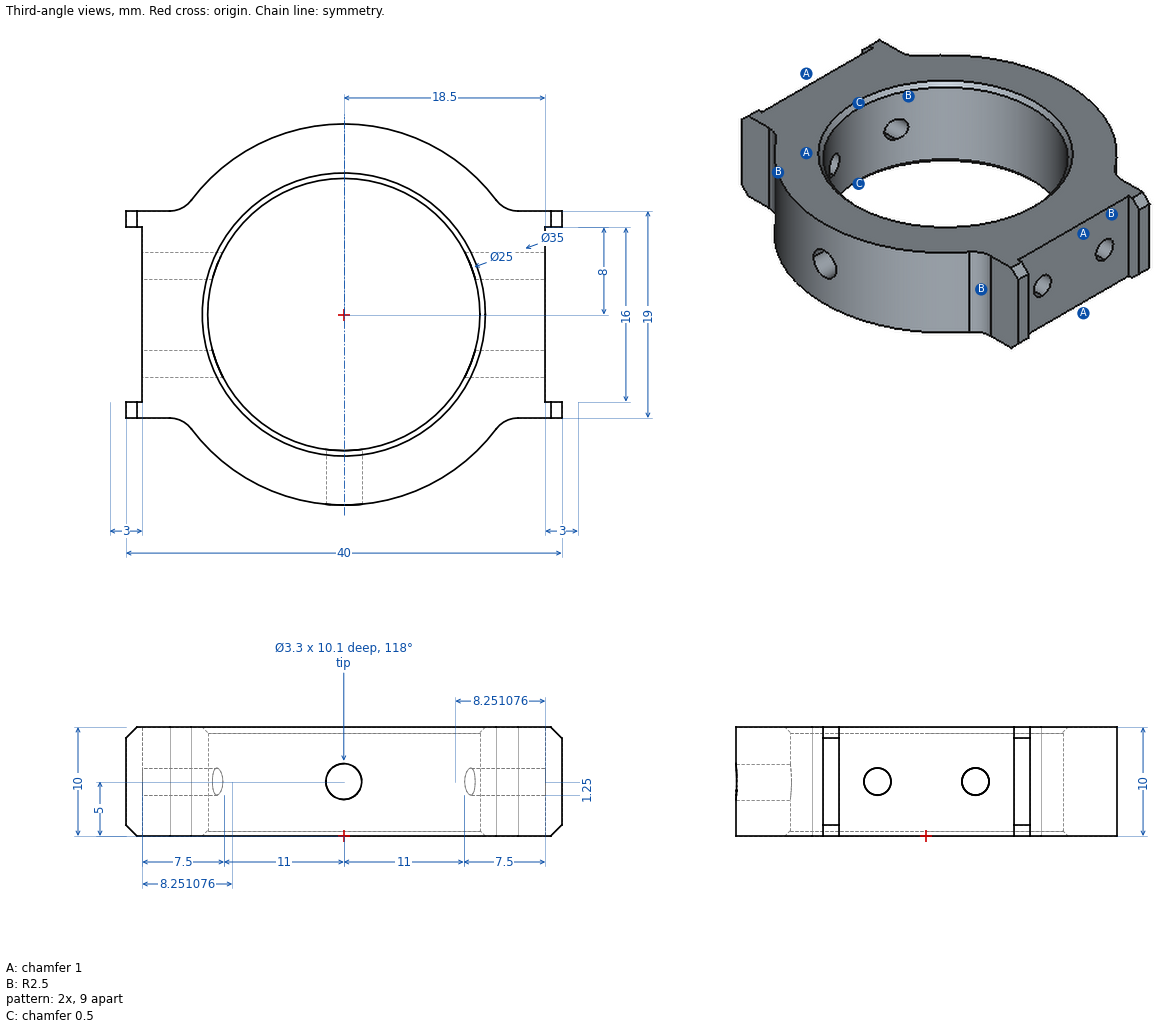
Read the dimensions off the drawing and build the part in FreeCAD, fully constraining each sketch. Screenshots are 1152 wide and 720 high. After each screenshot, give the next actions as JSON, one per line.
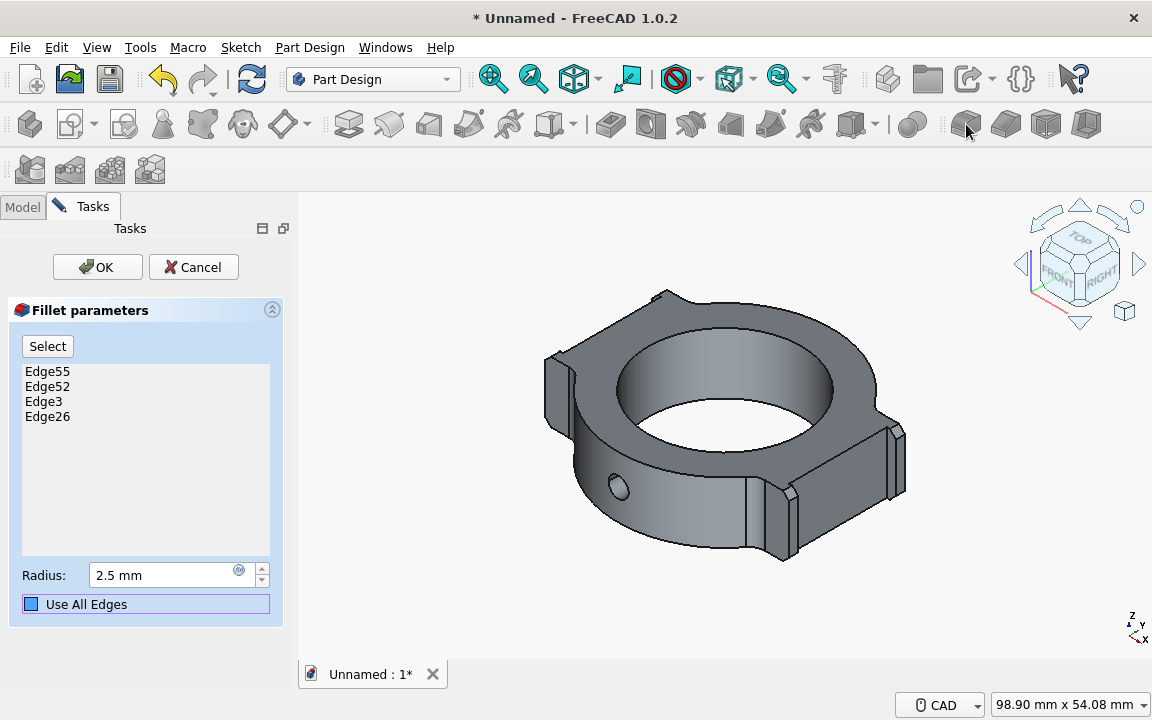
{"action": "left_click", "coordinate": [98, 267]}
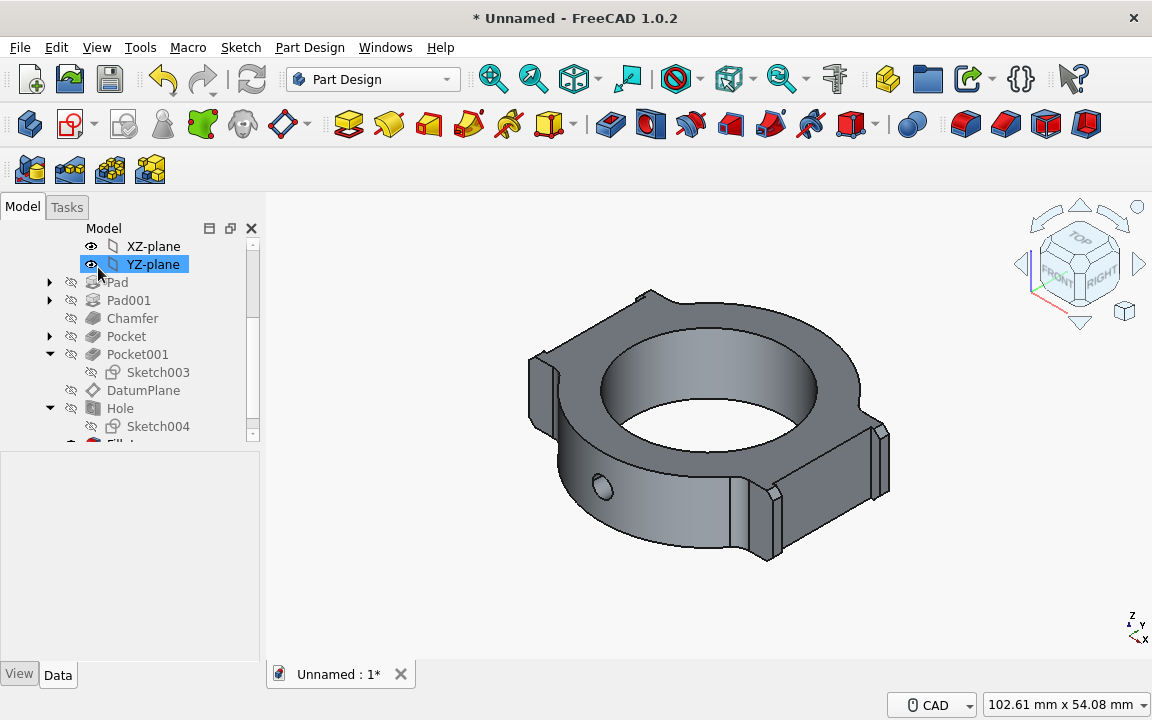
{"action": "scroll", "coordinate": [160, 332], "scroll_direction": "down", "scroll_amount": 3}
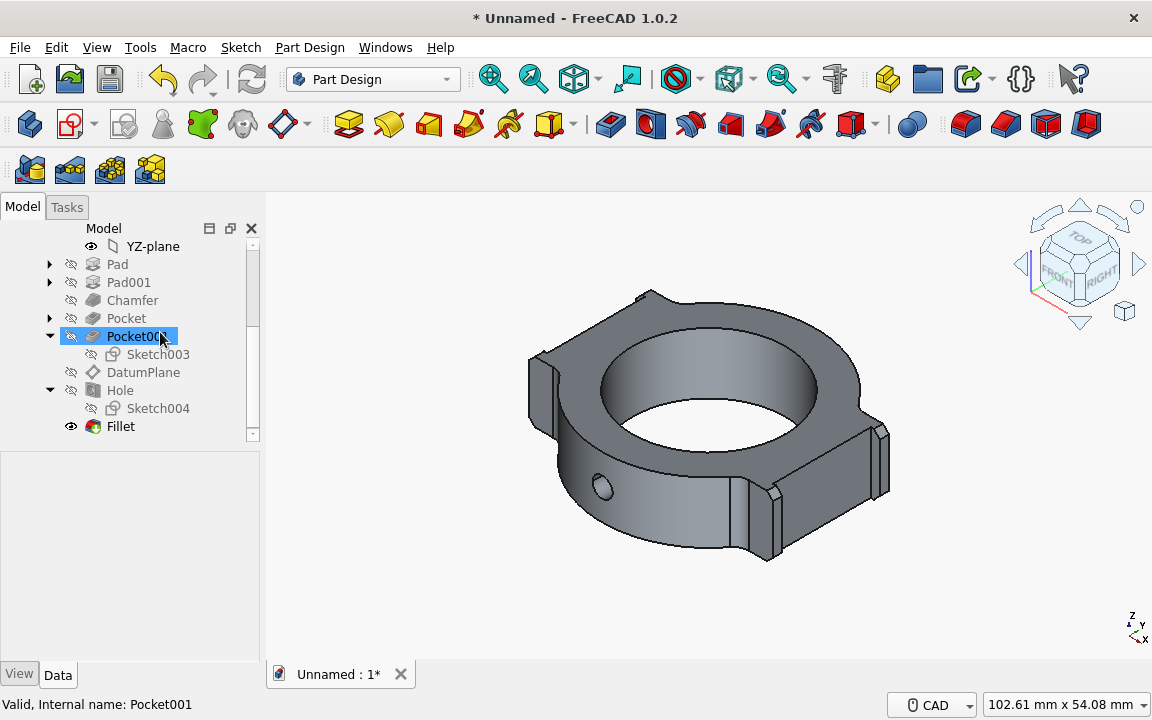
{"action": "scroll", "coordinate": [160, 332], "scroll_direction": "up", "scroll_amount": 15}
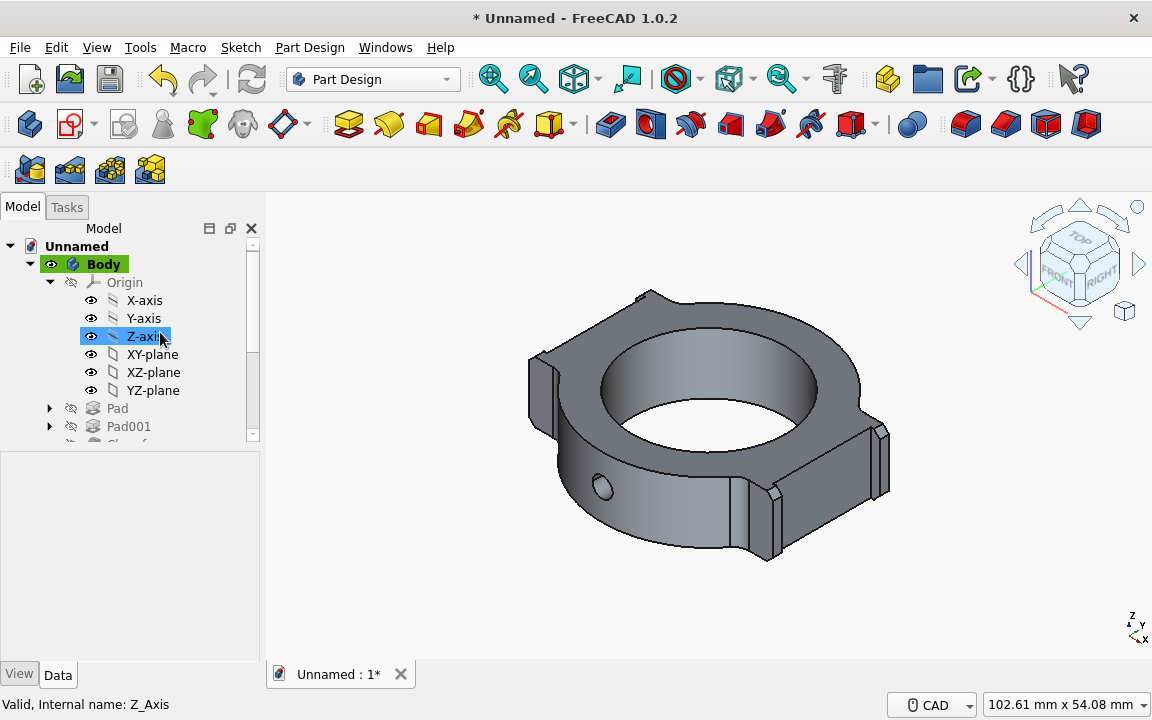
{"action": "left_click", "coordinate": [136, 372]}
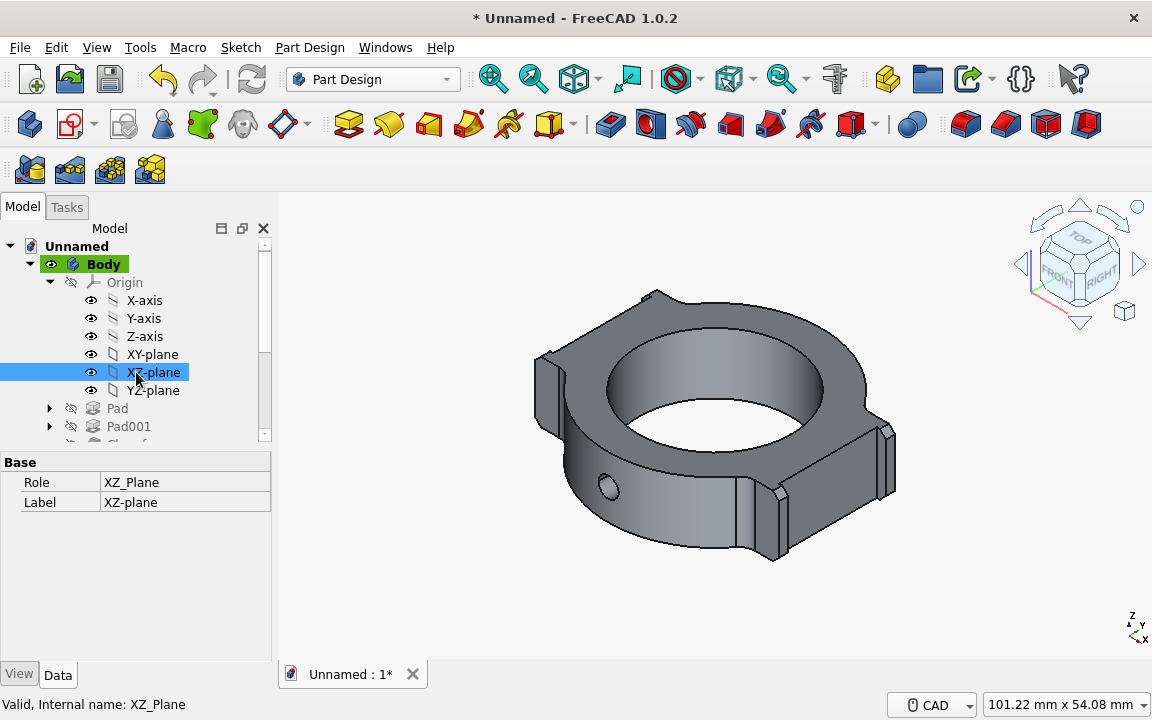
{"action": "left_click", "coordinate": [284, 124]}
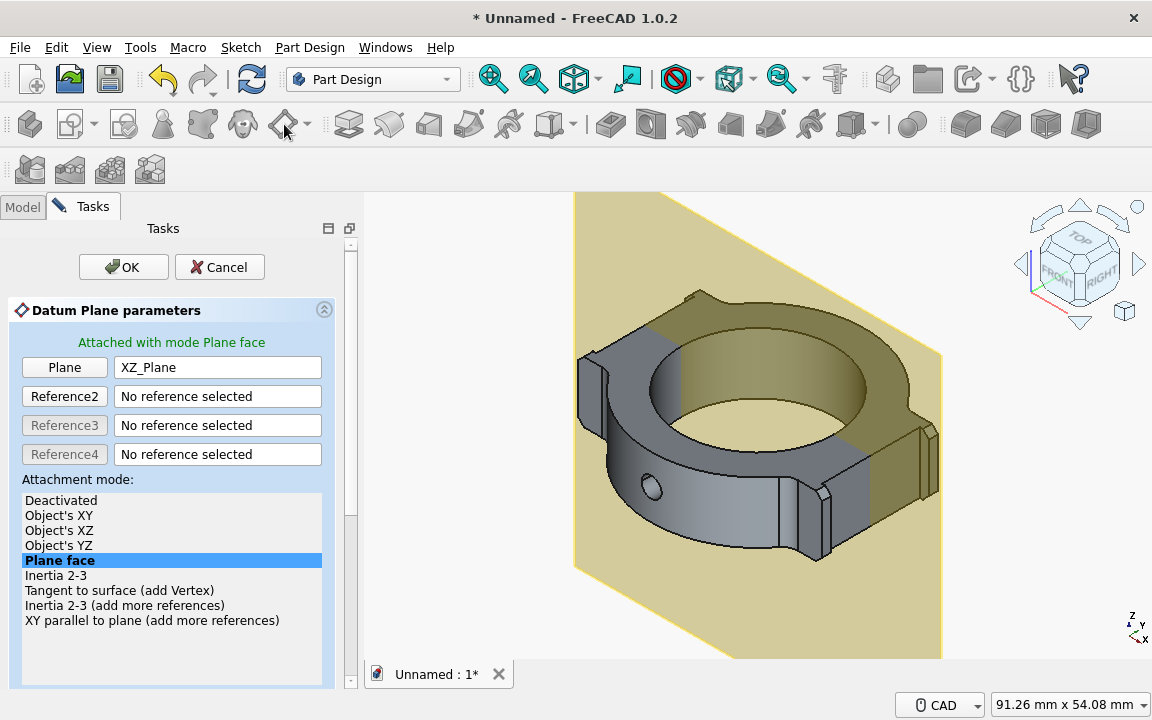
{"action": "scroll", "coordinate": [351, 463], "scroll_direction": "down", "scroll_amount": 3}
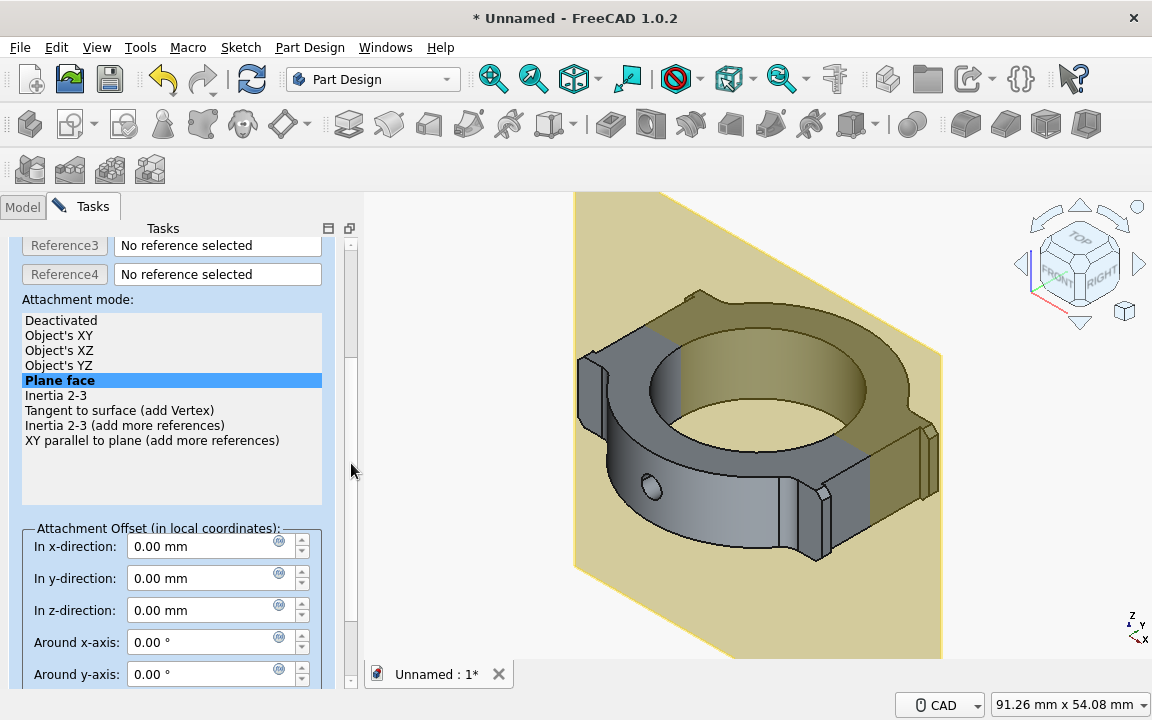
{"action": "triple_click", "coordinate": [210, 610]}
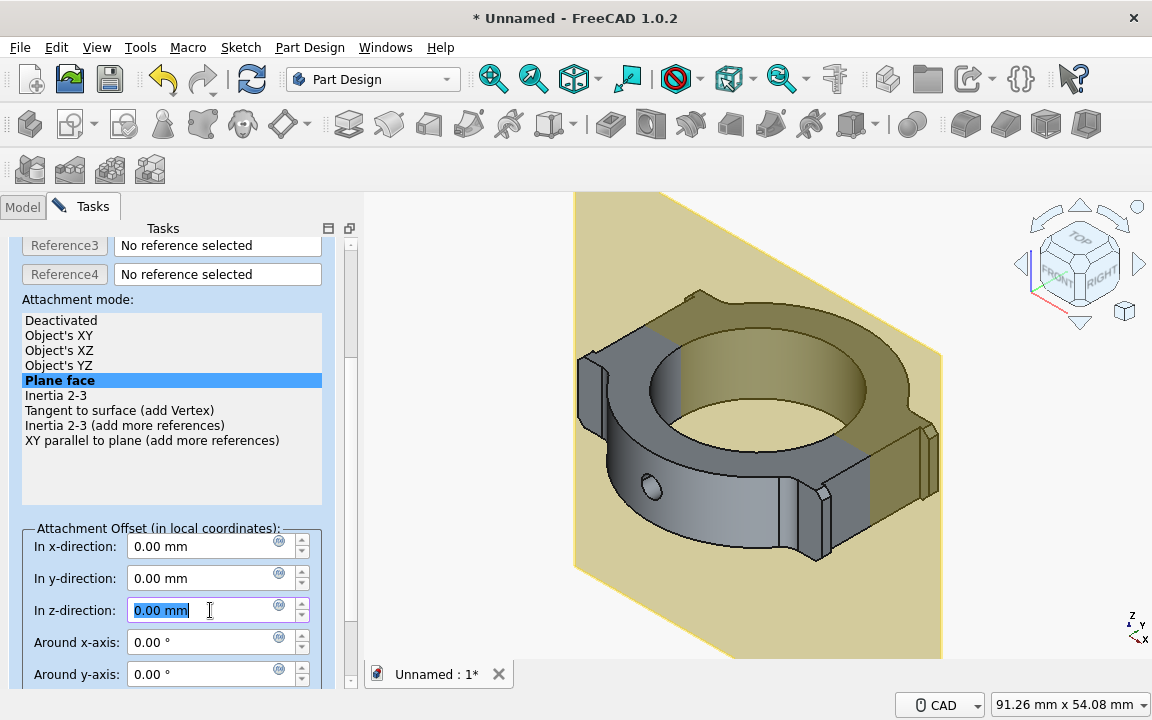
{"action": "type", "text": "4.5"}
{"action": "key", "text": "Tab"}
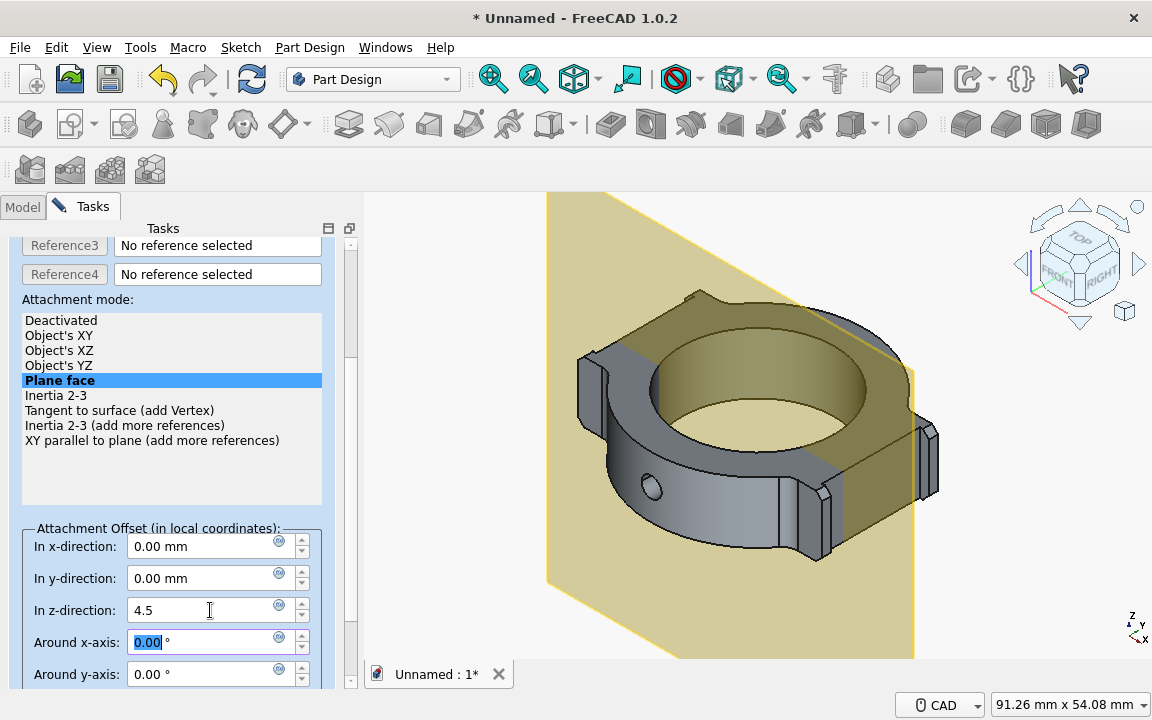
{"action": "scroll", "coordinate": [351, 463], "scroll_direction": "up", "scroll_amount": 4}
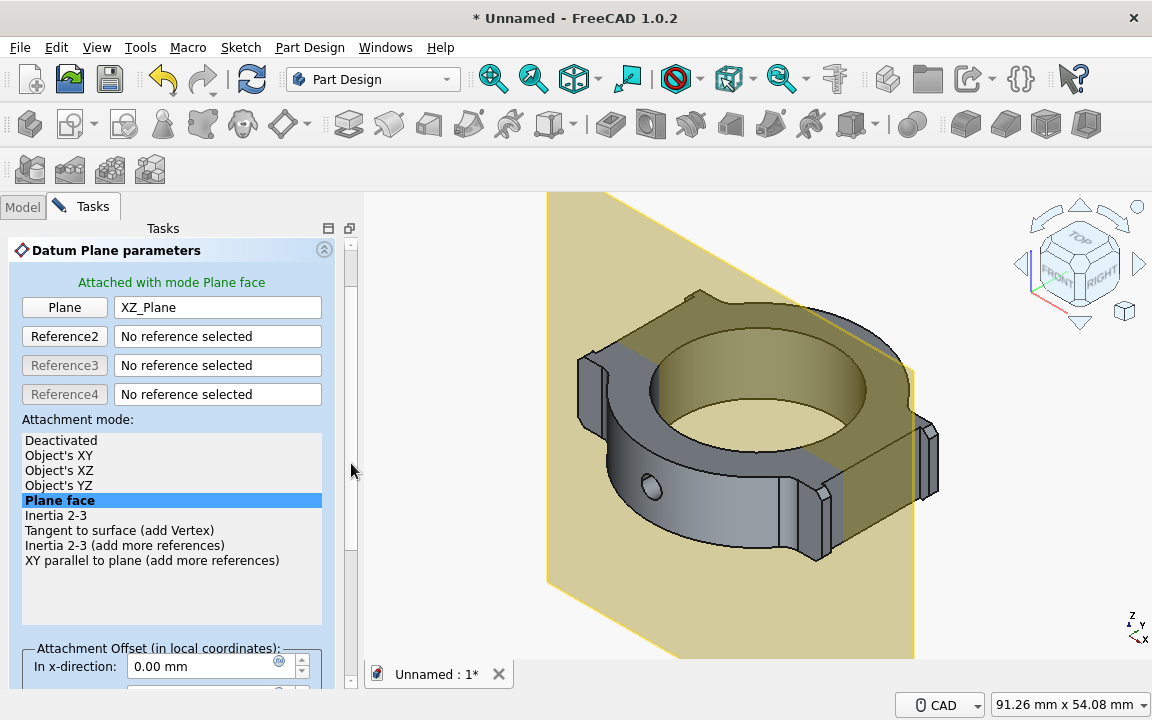
{"action": "left_click", "coordinate": [124, 267]}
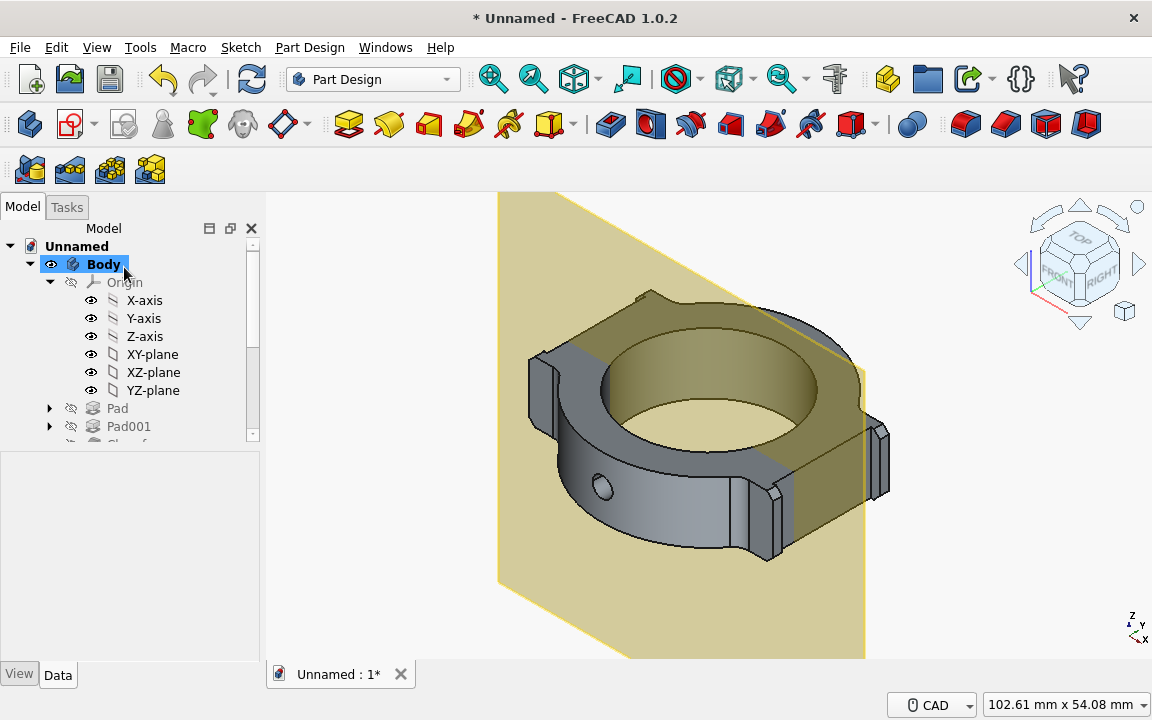
{"action": "scroll", "coordinate": [100, 332], "scroll_direction": "down", "scroll_amount": 3}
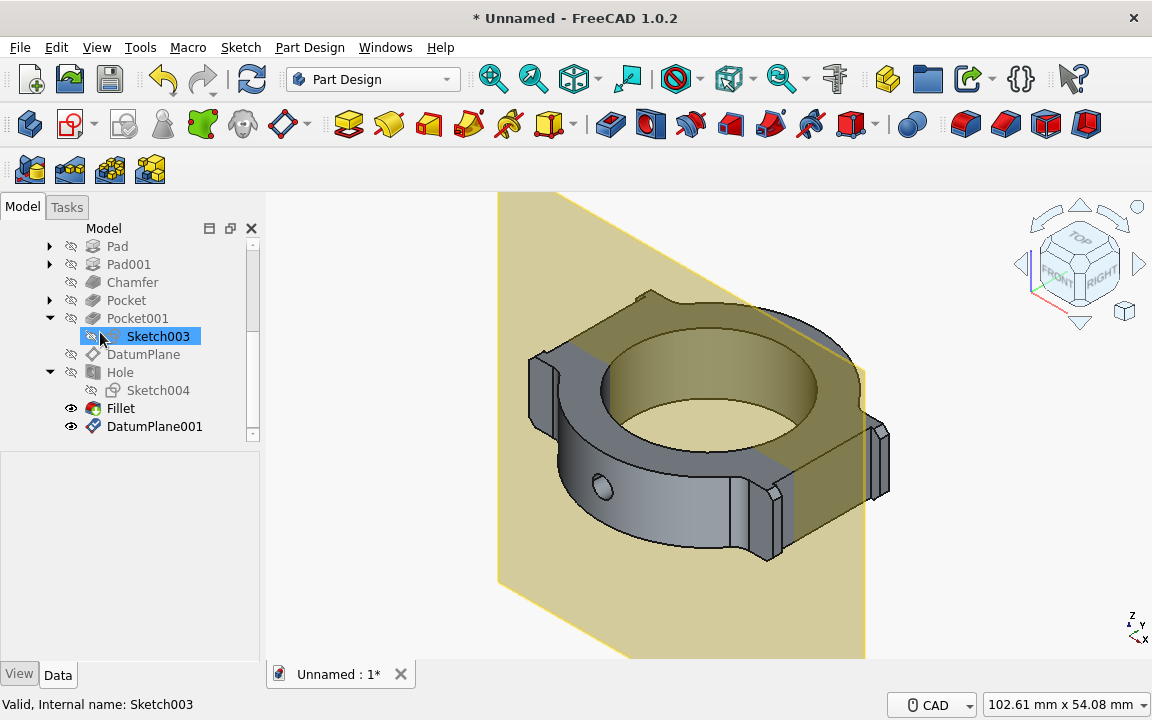
{"action": "left_click", "coordinate": [116, 426]}